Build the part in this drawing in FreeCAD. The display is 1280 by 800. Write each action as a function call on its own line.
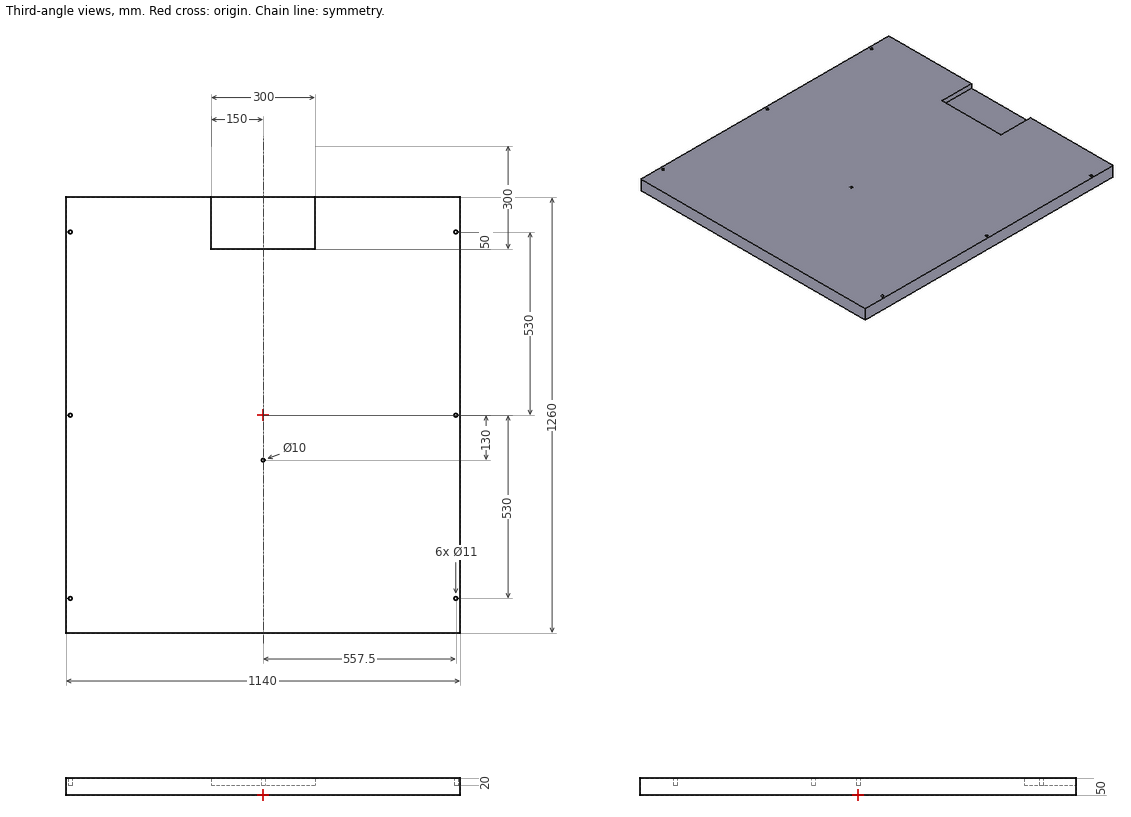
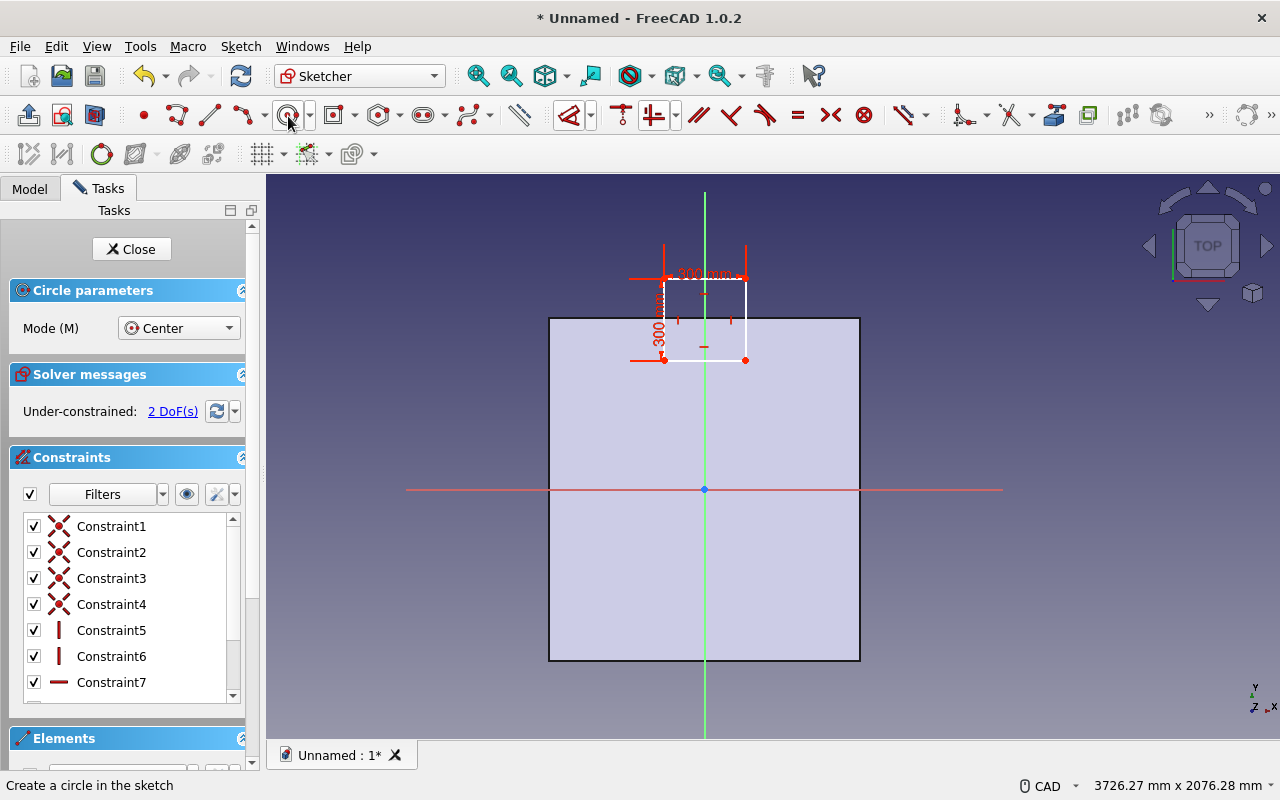
scroll(705, 525, up, 15)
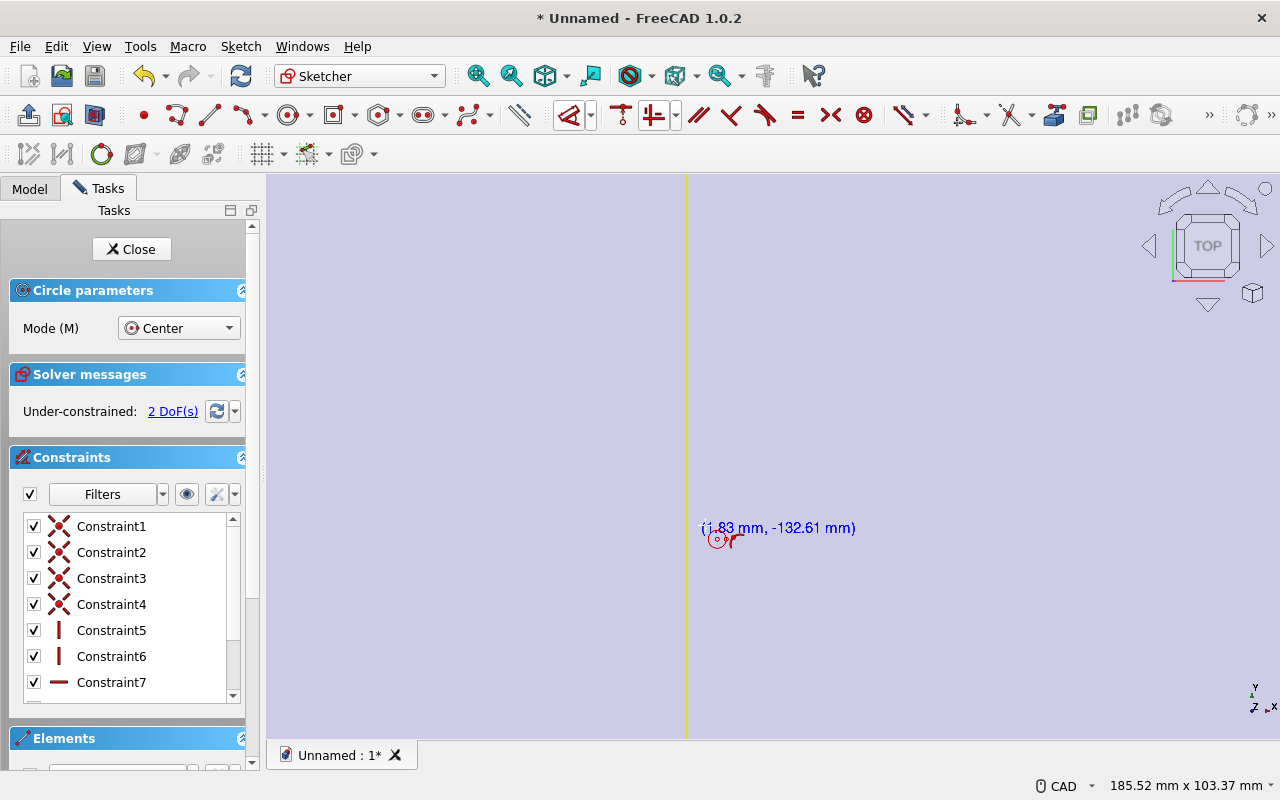
scroll(705, 525, down, 15)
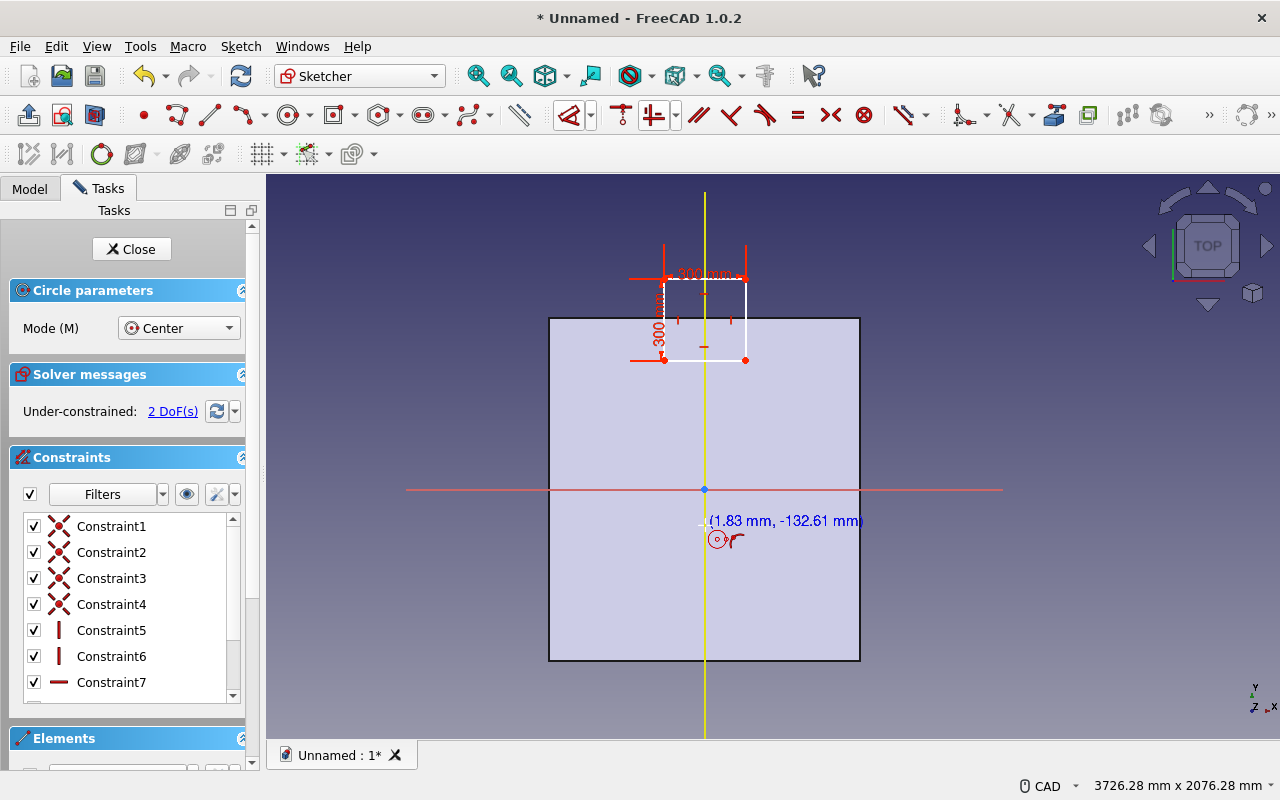
click(705, 525)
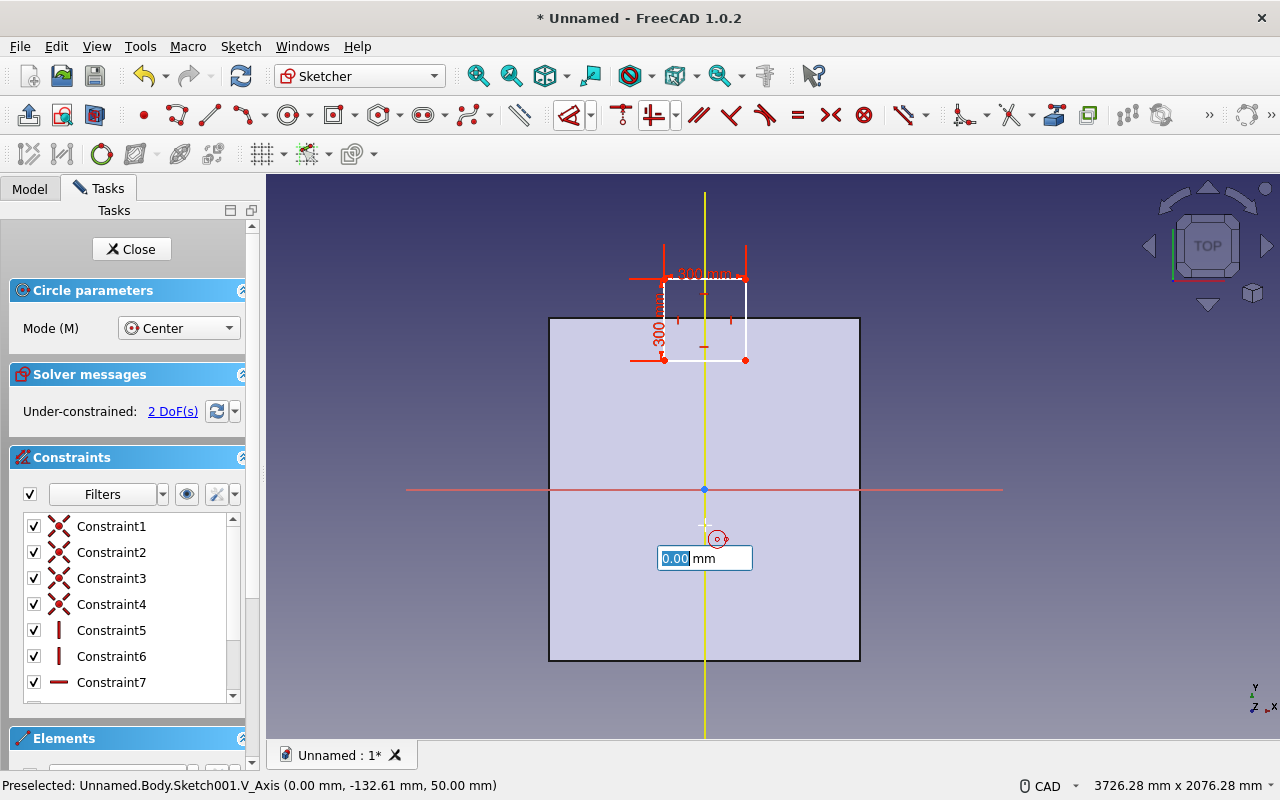
scroll(706, 525, up, 13)
move(698, 515)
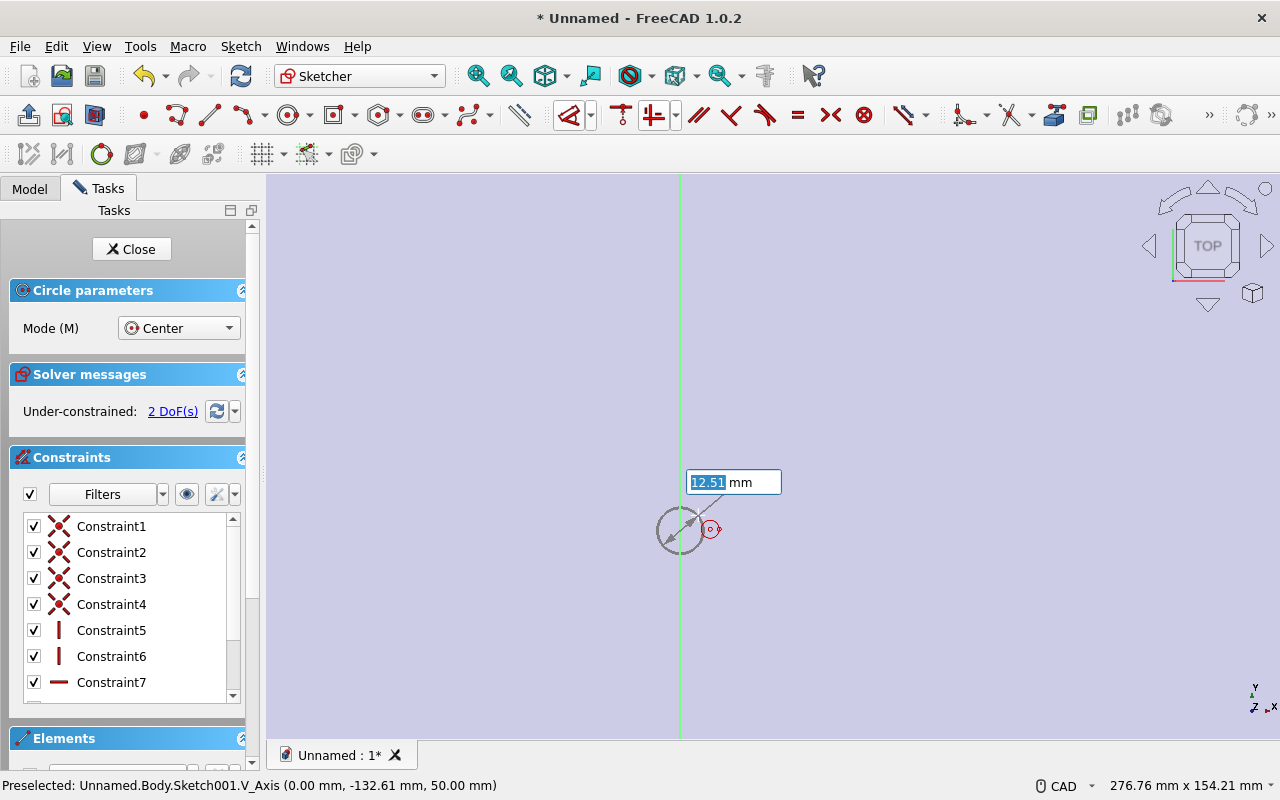
text(10)
key(Return)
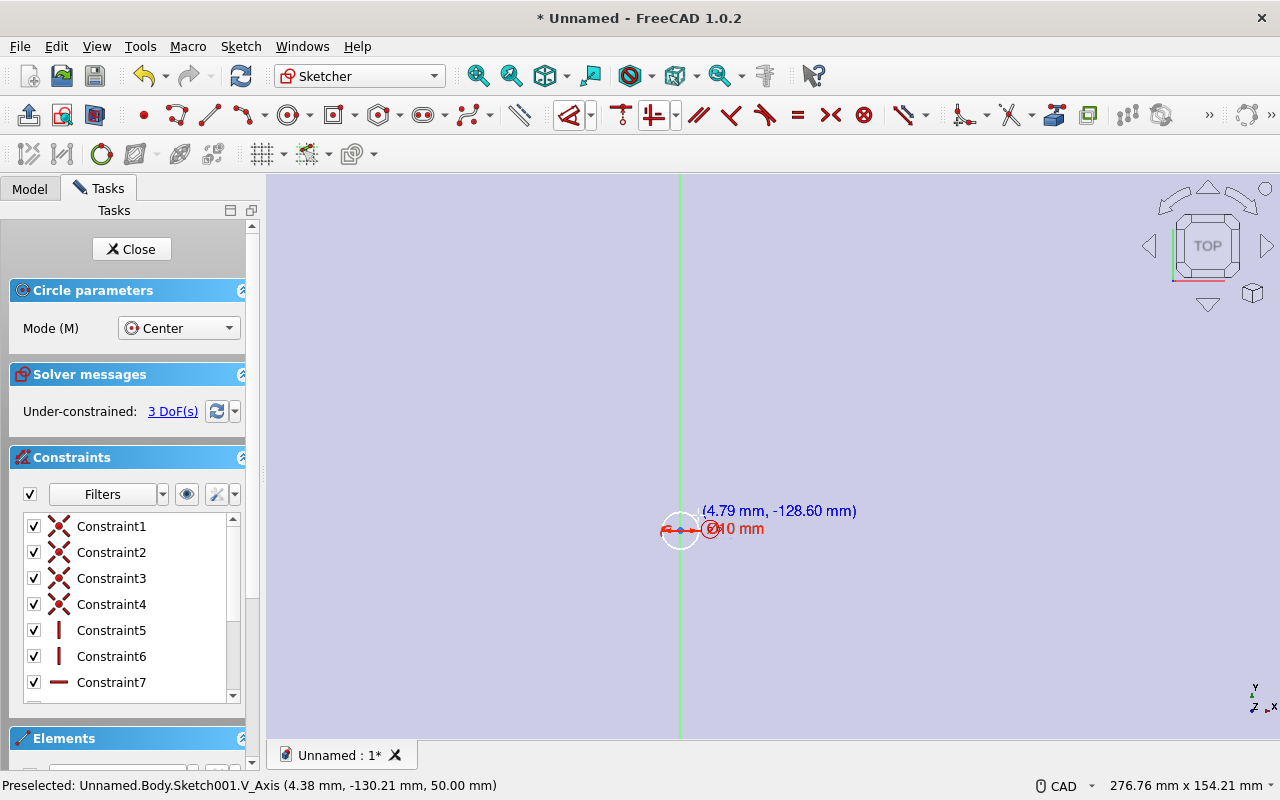
scroll(706, 525, down, 13)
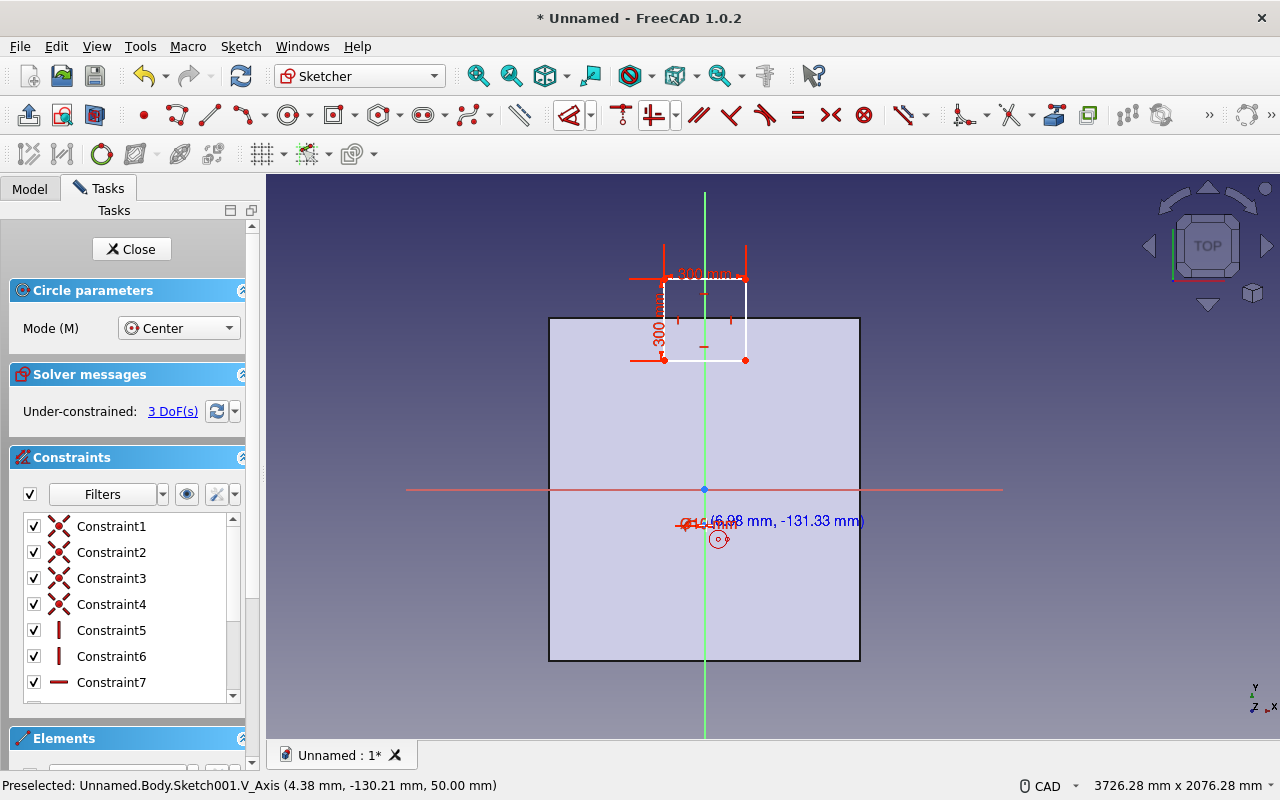
scroll(856, 634, up, 14)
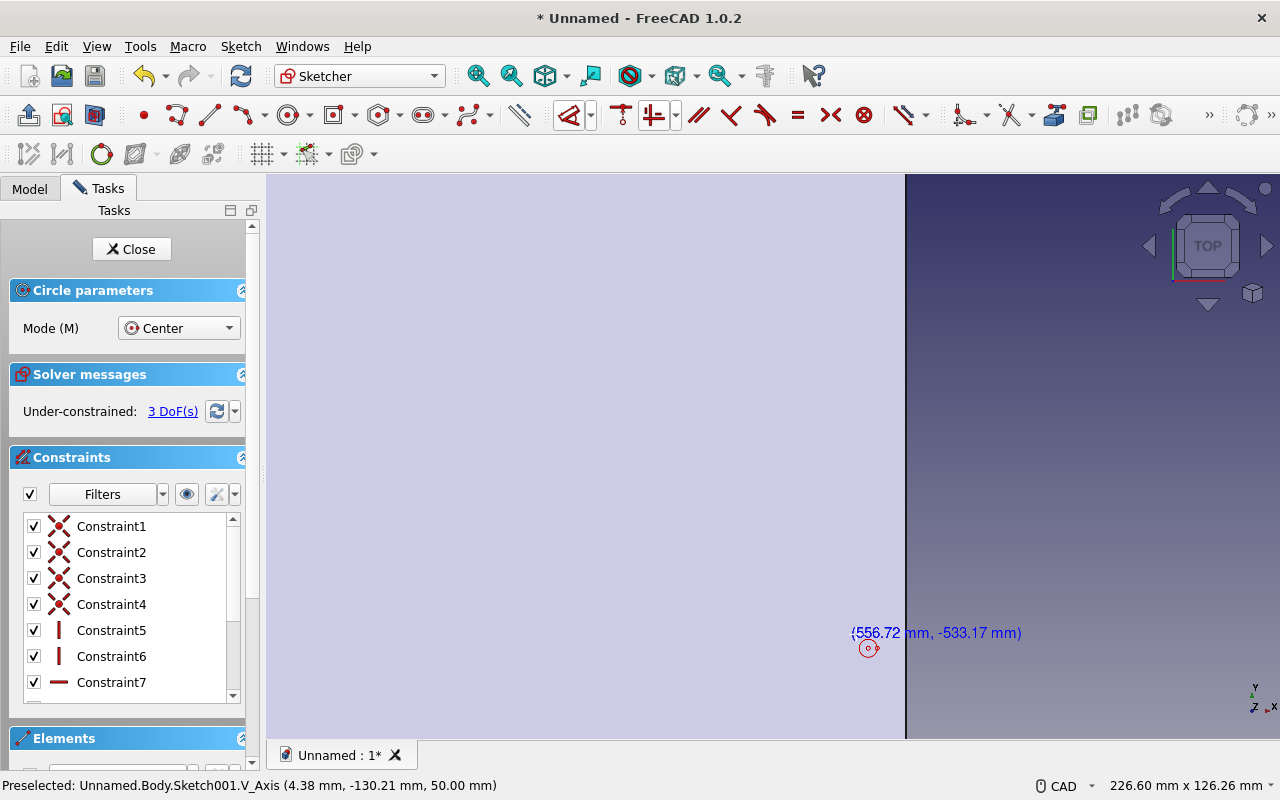
scroll(857, 635, down, 14)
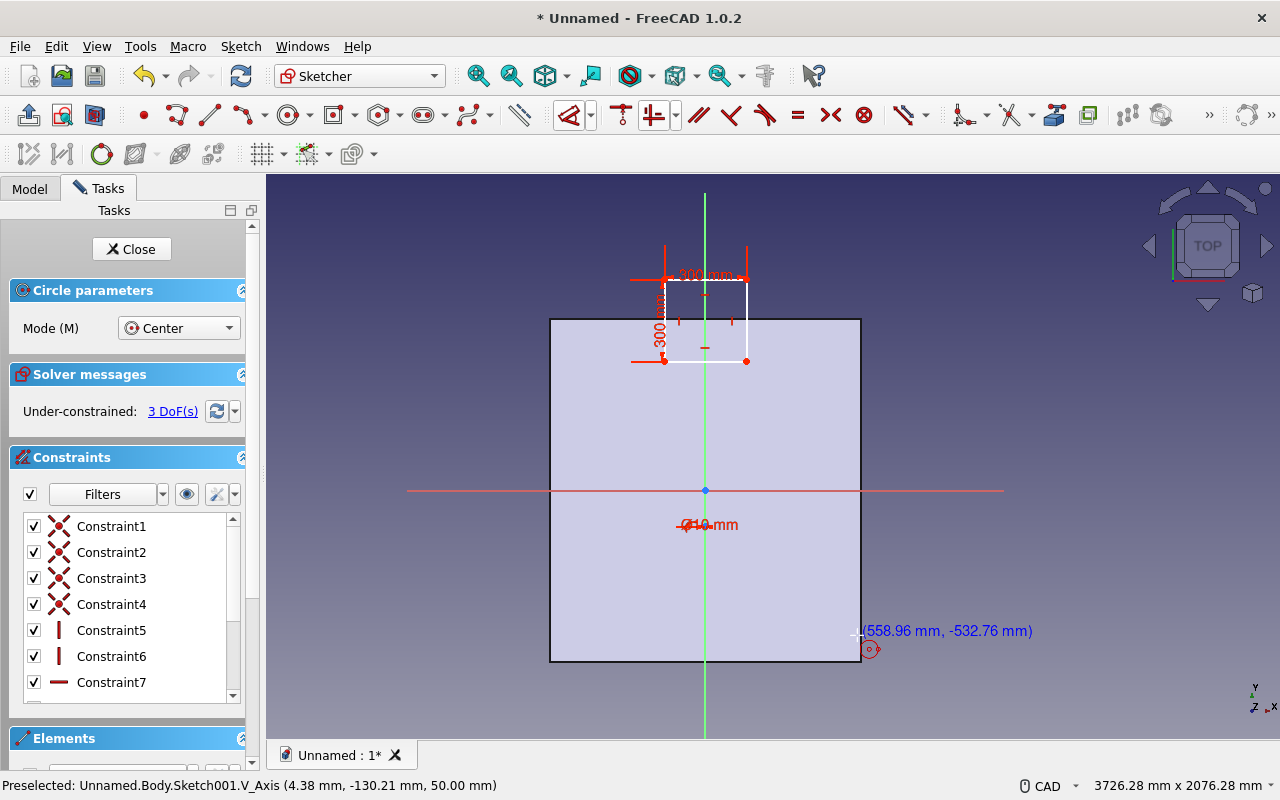
click(857, 635)
move(858, 634)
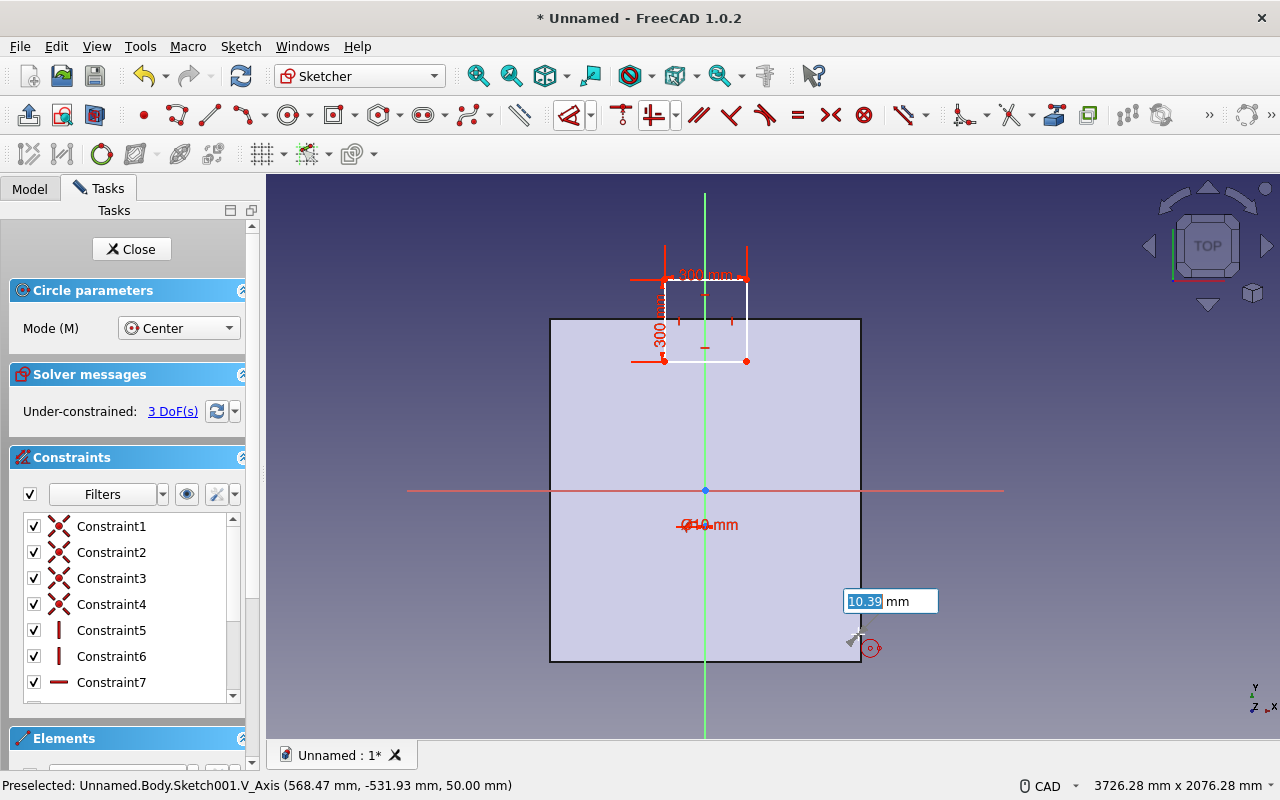
text(11)
key(Return)